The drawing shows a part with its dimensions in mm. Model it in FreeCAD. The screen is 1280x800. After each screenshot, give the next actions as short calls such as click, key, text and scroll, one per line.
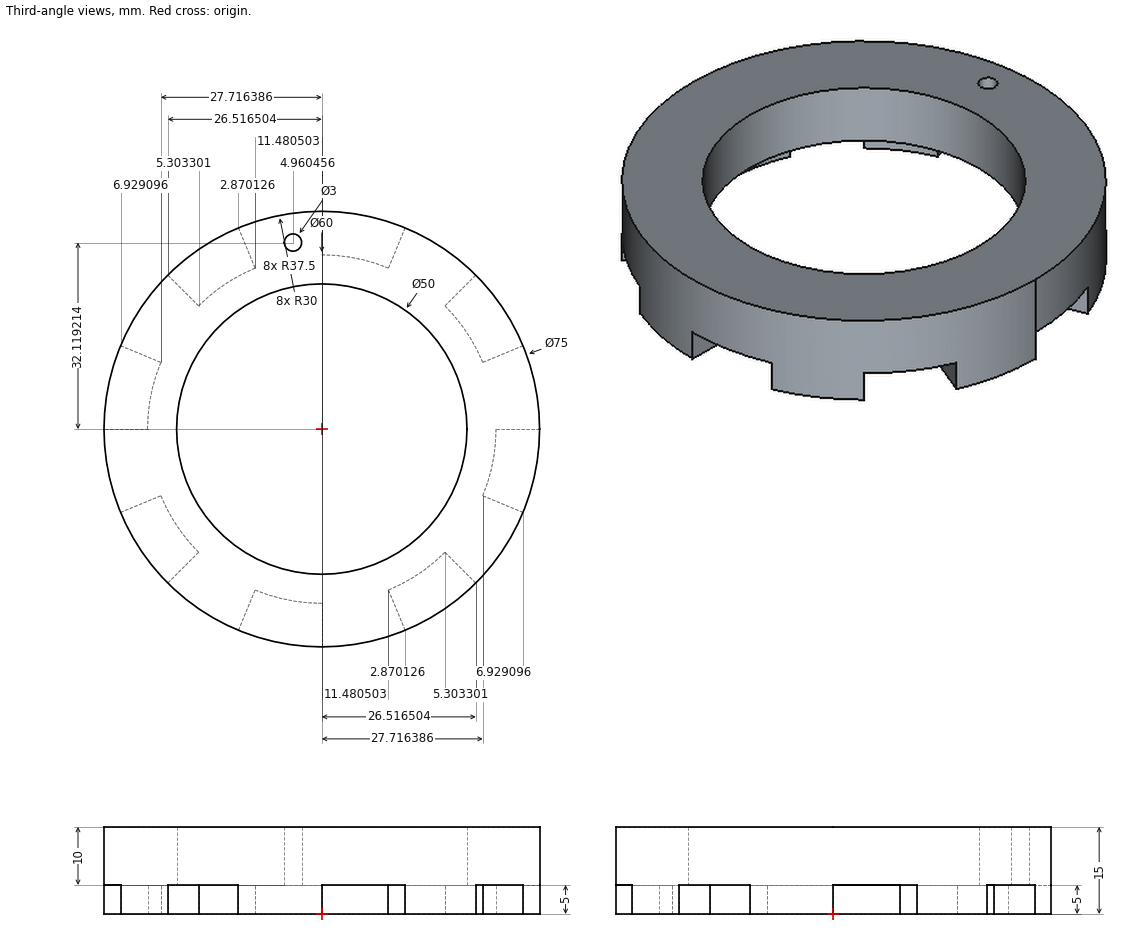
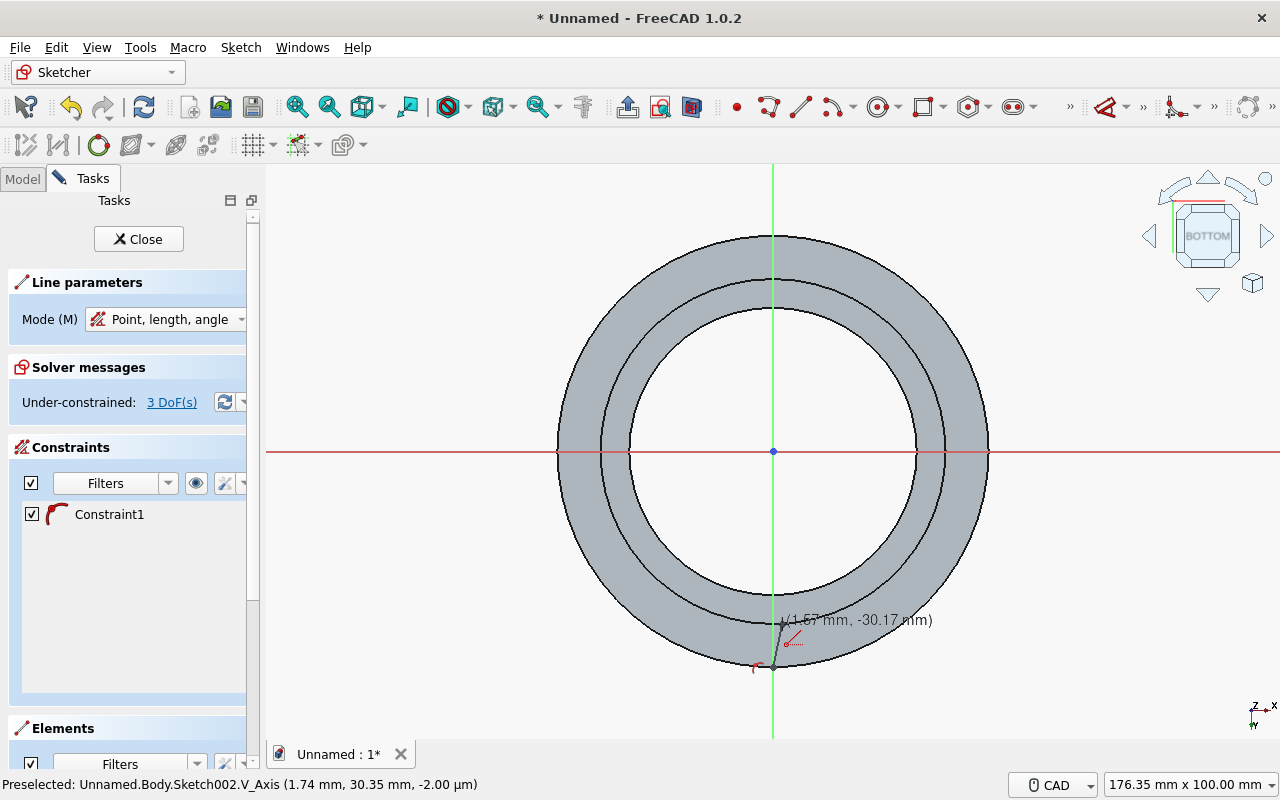
click(707, 611)
click(690, 651)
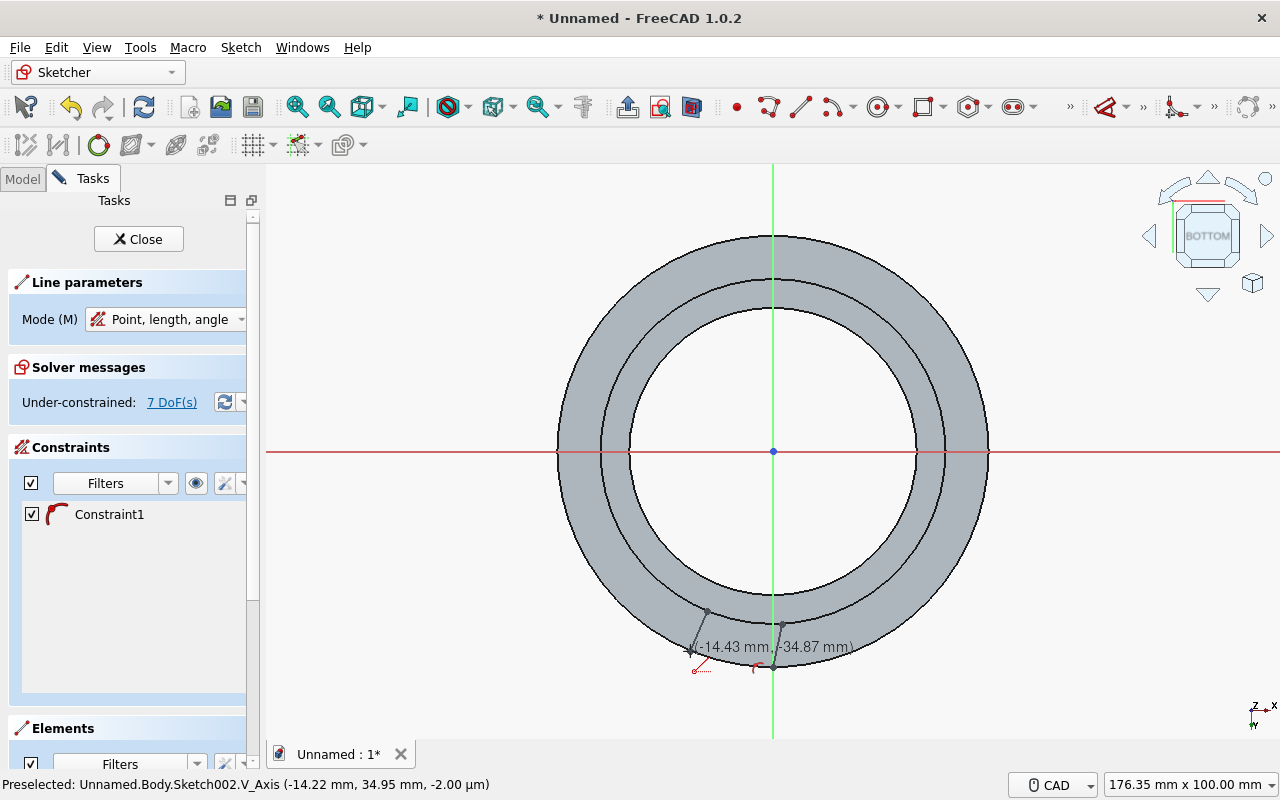
key(g)
key(3)
key(a)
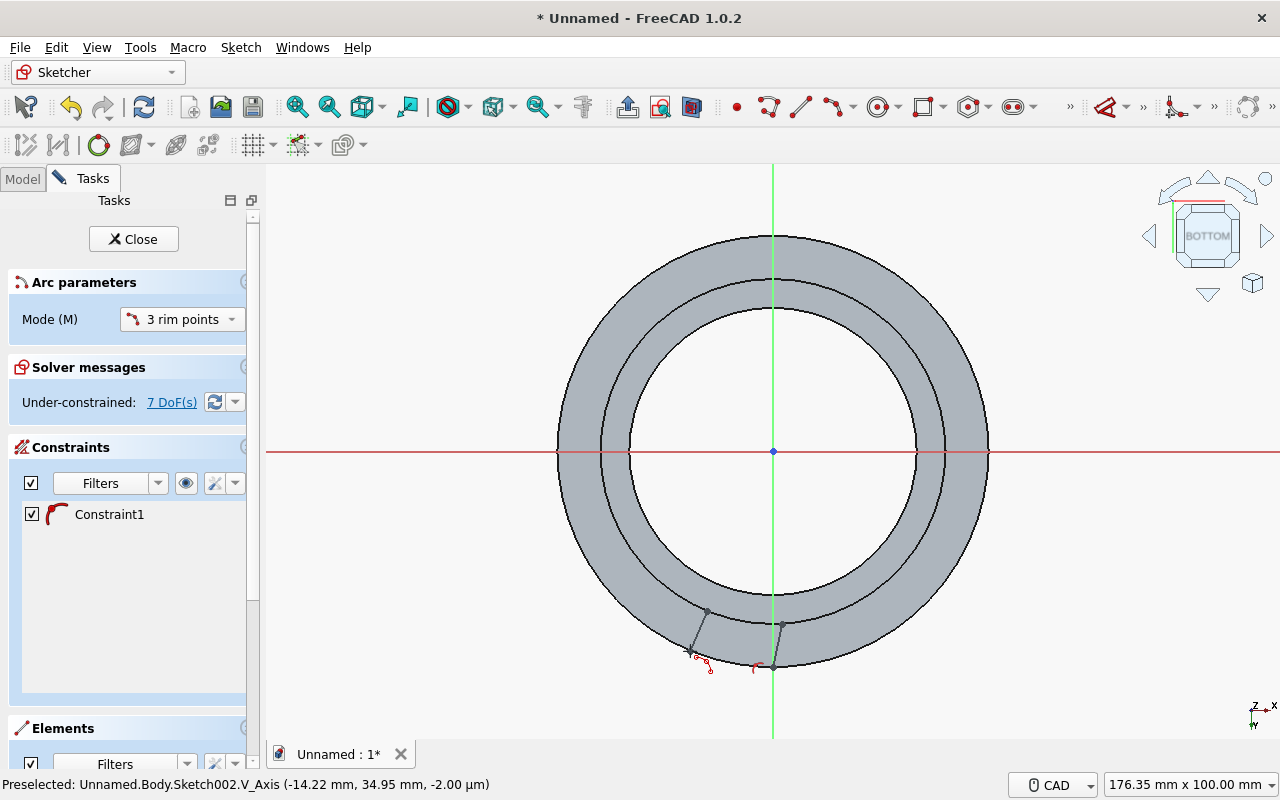
click(782, 625)
click(707, 612)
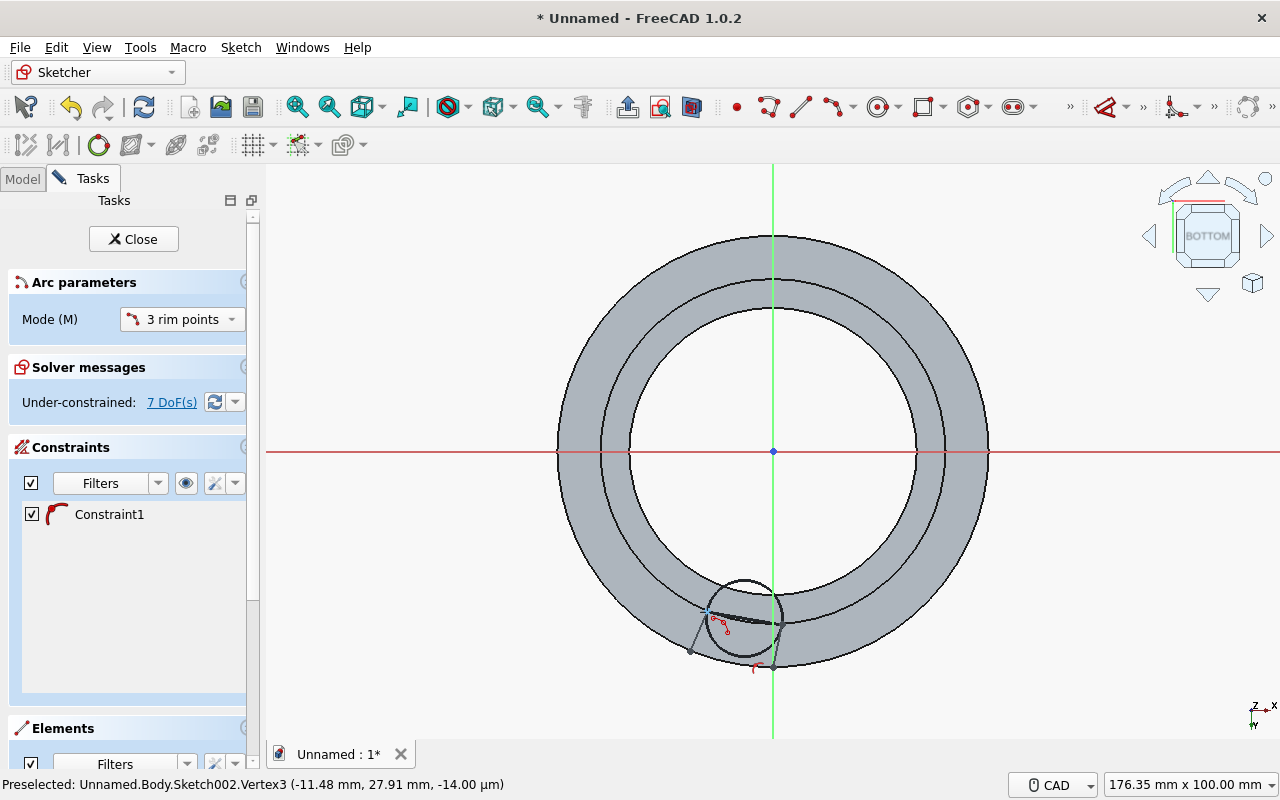
scroll(739, 621, up, 8)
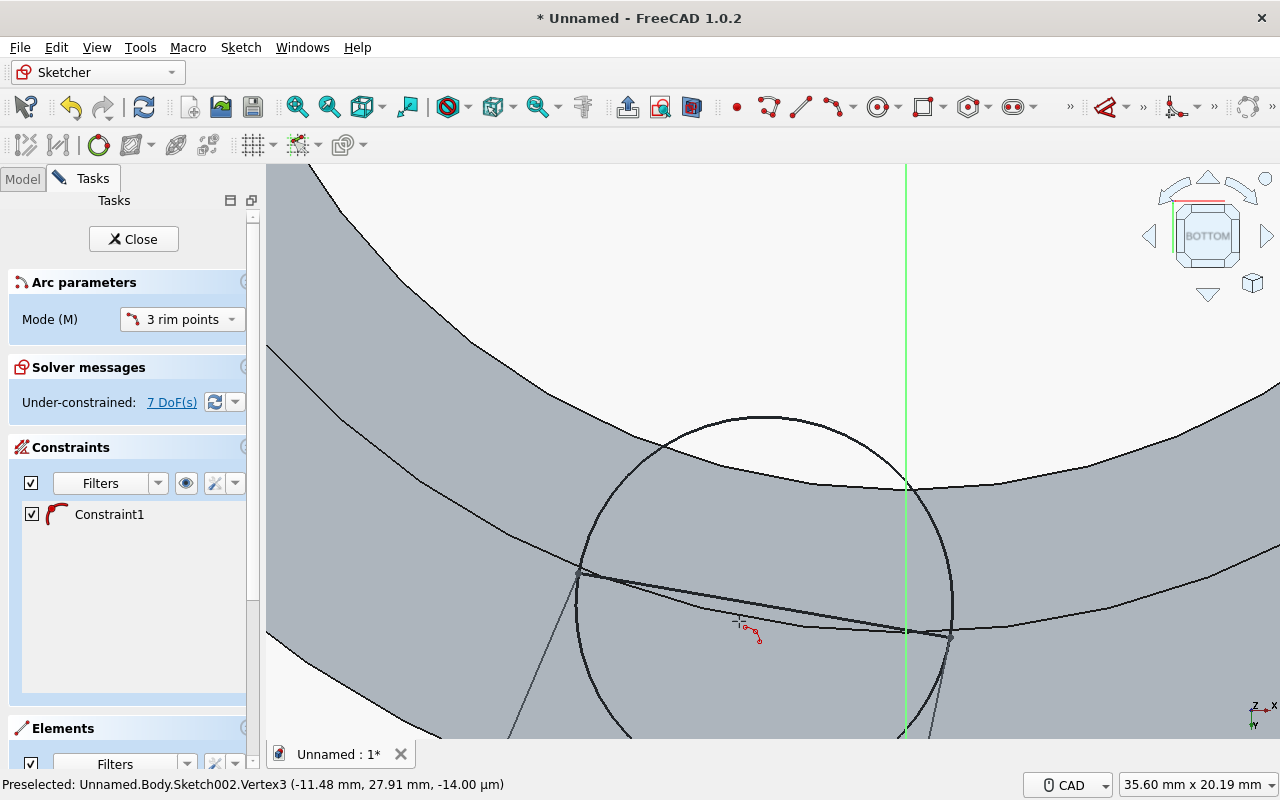
click(739, 616)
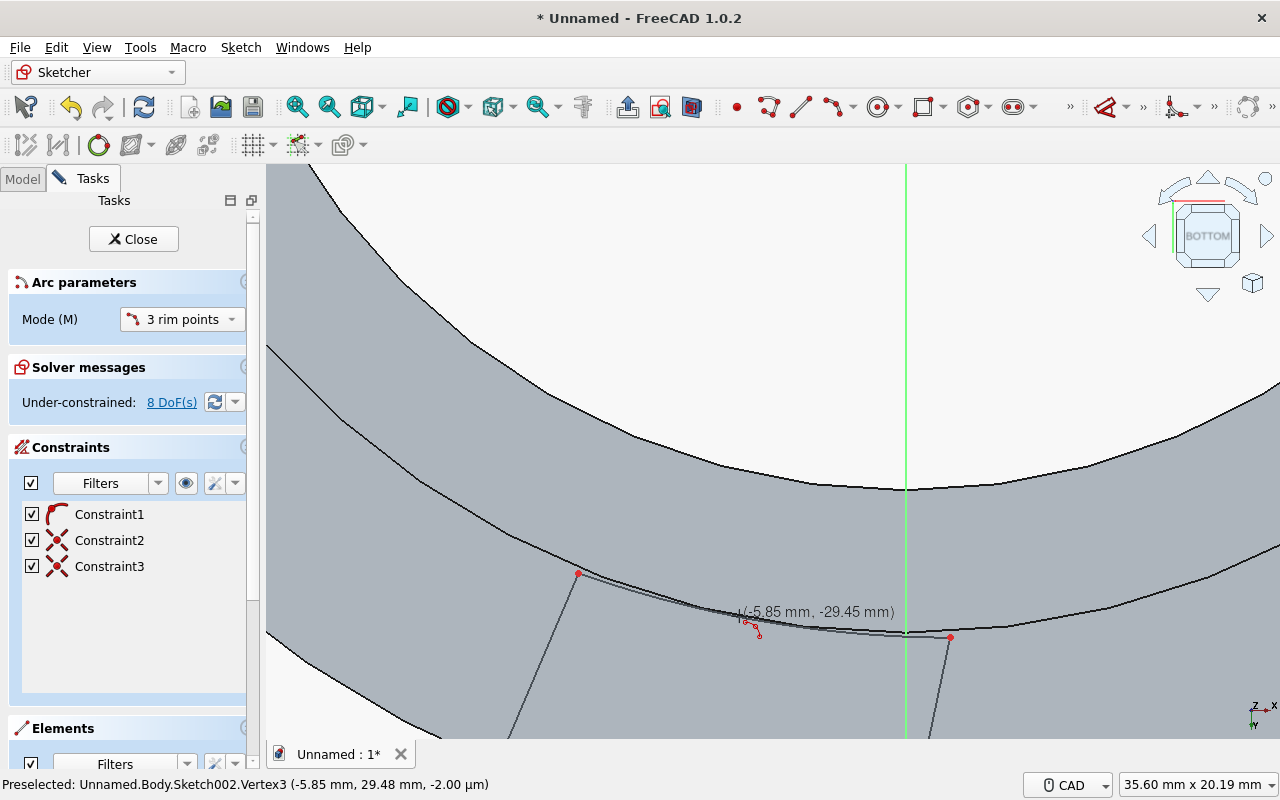
scroll(665, 585, down, 9)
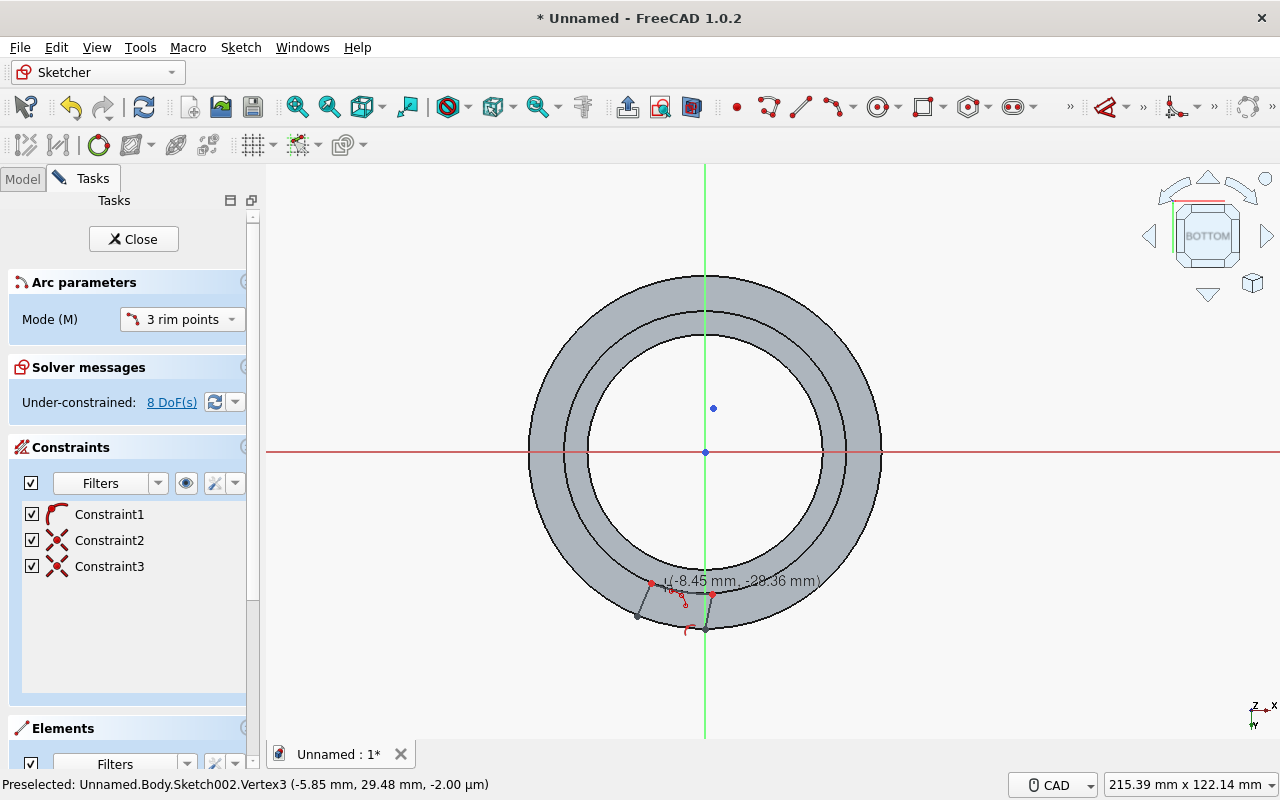
click(637, 616)
click(705, 630)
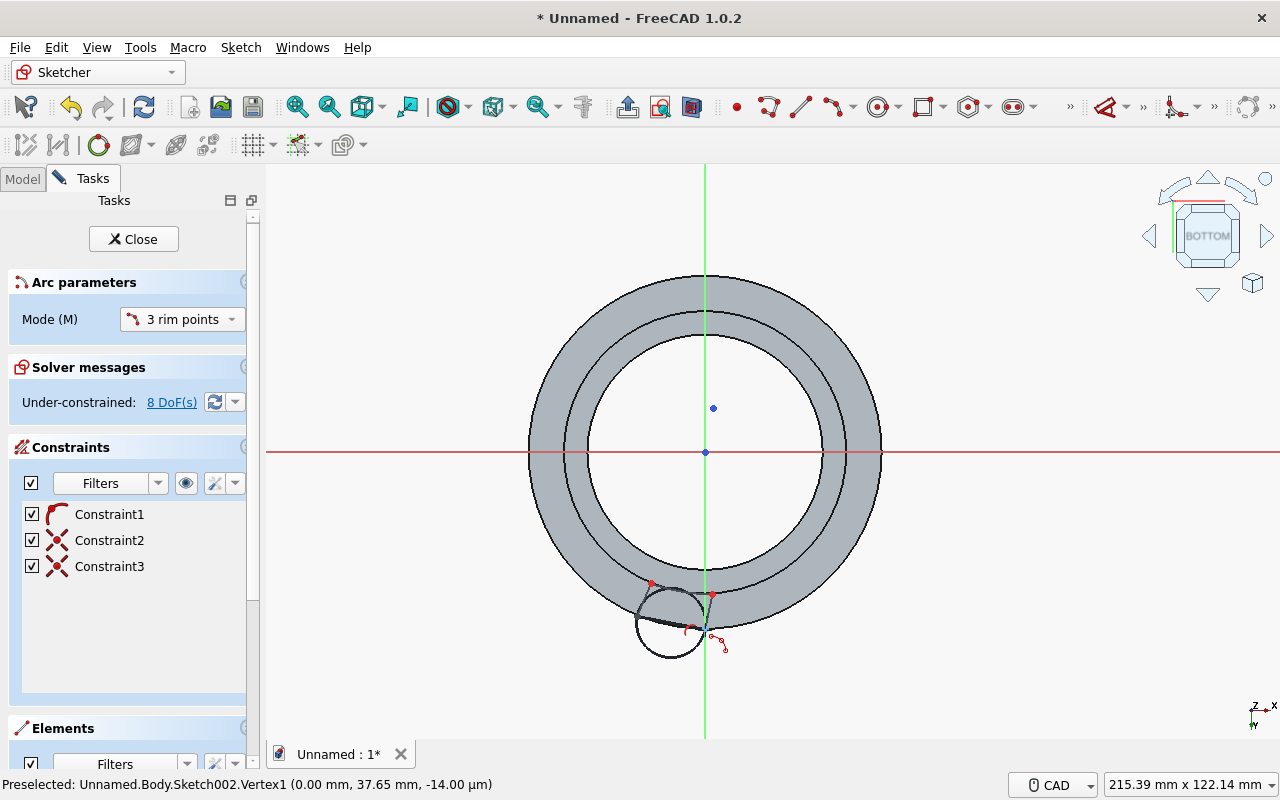
scroll(671, 625, up, 8)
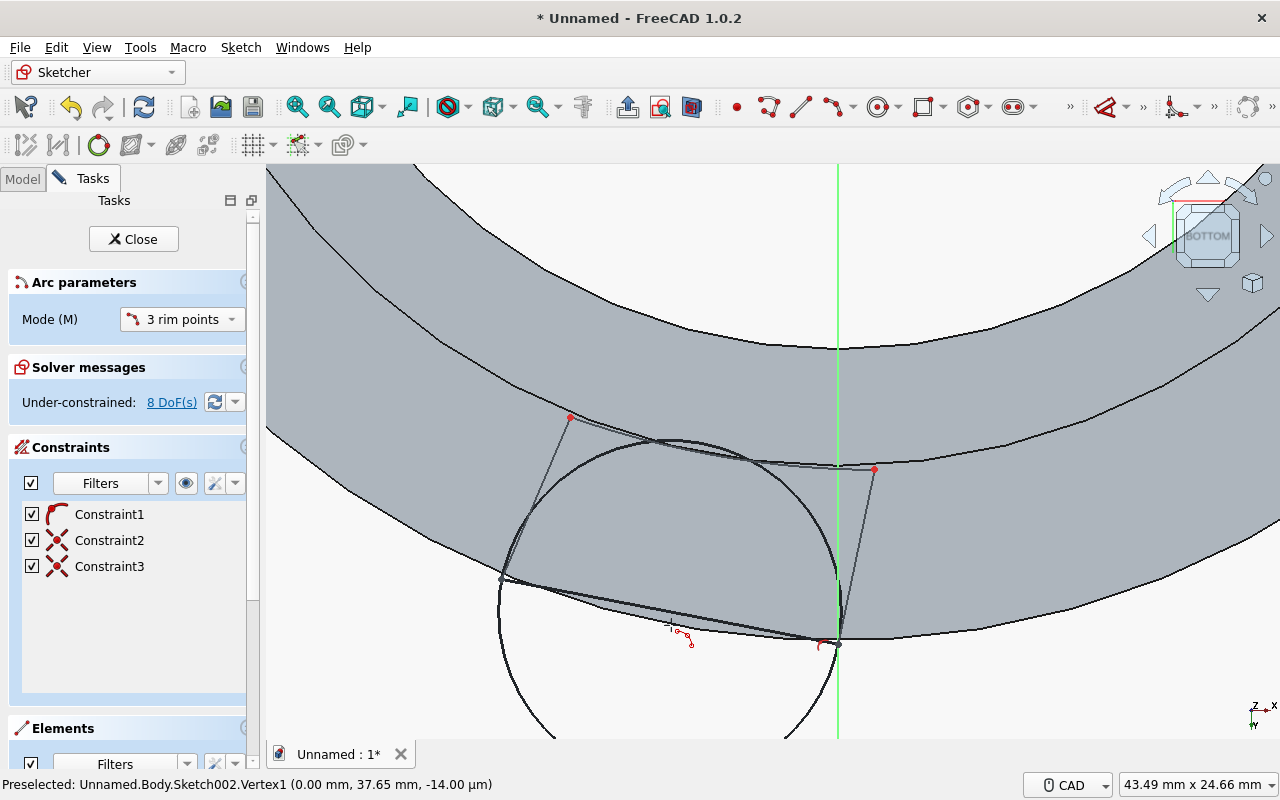
click(668, 624)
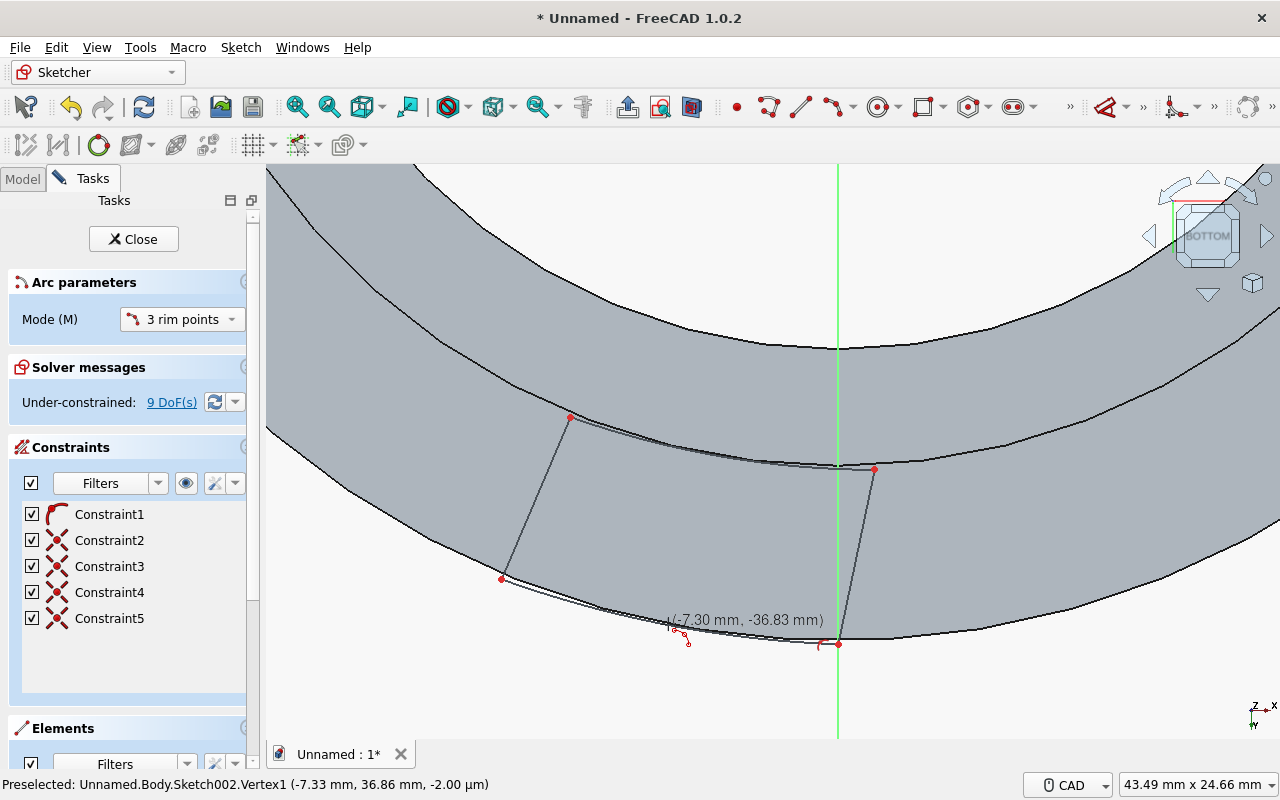
click(802, 108)